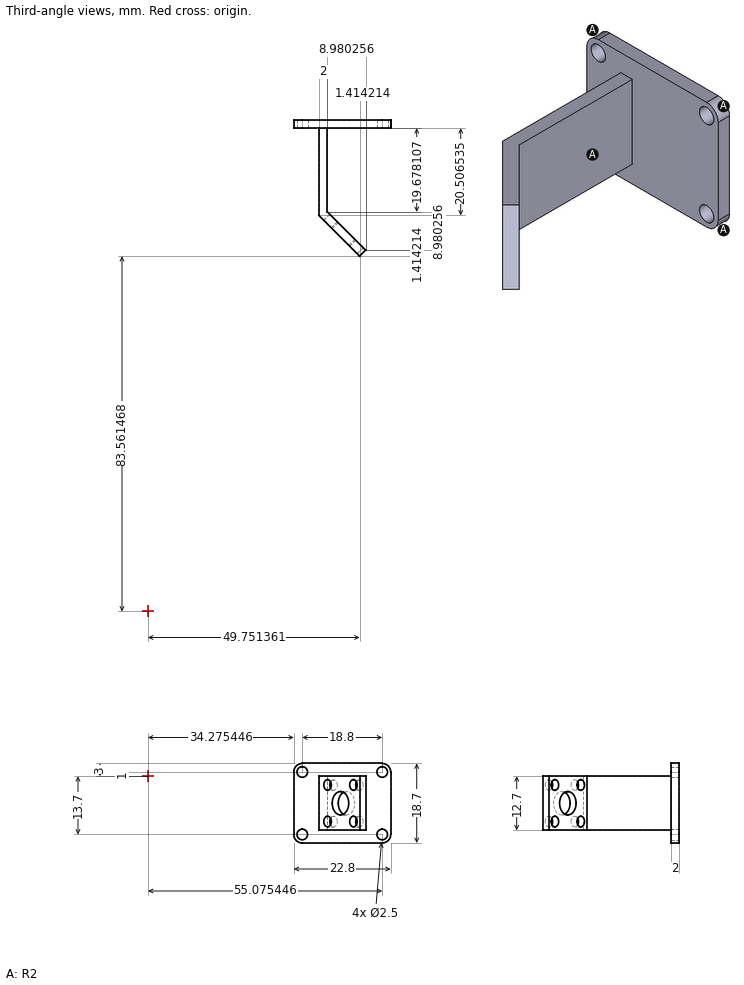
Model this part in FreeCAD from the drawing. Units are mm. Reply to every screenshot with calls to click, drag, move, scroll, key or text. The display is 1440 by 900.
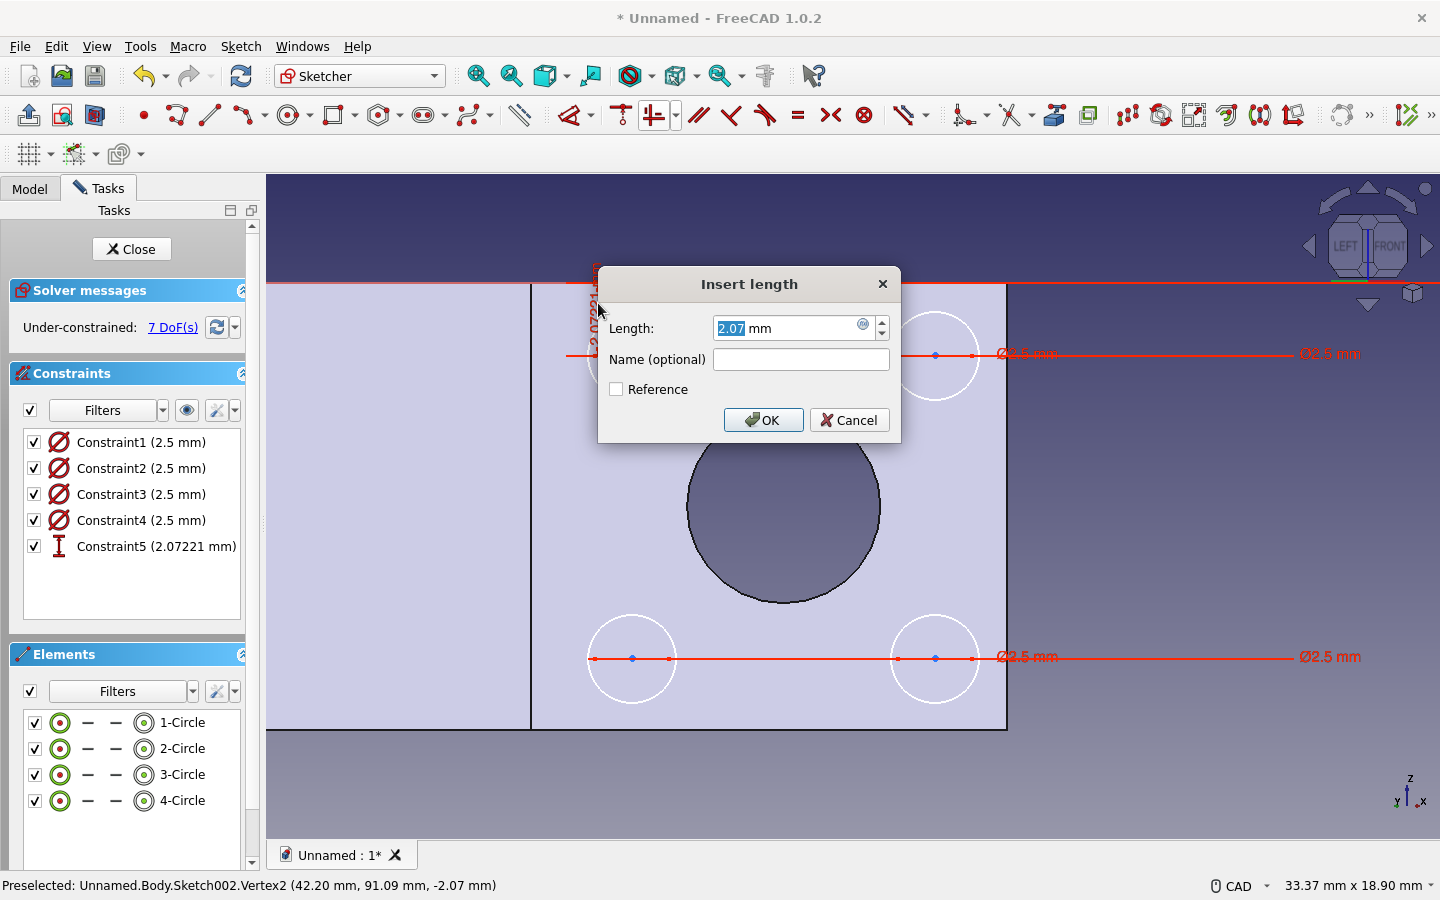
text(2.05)
key(Return)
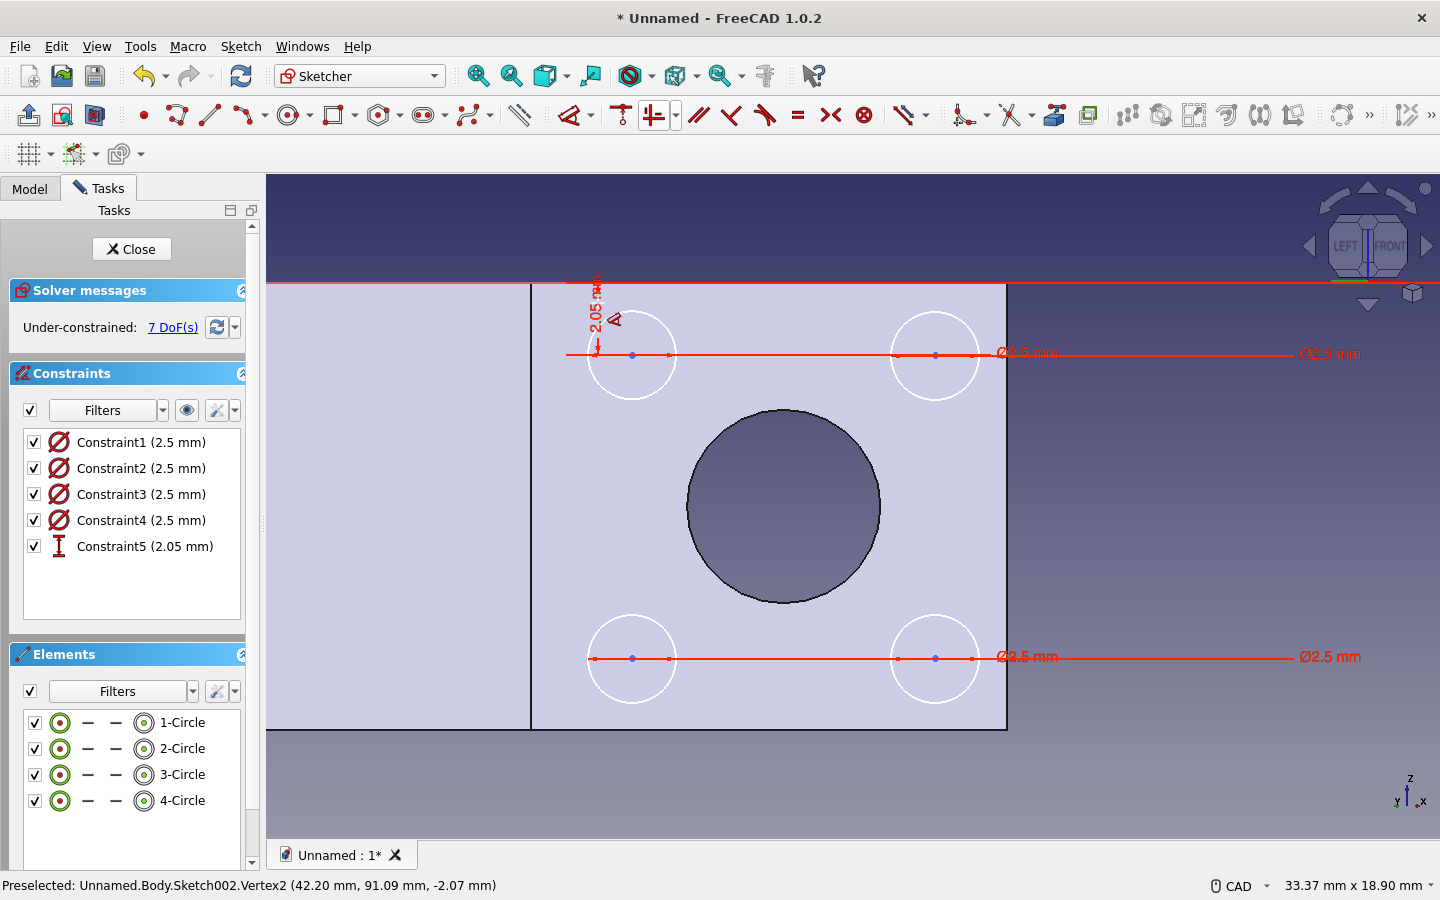
click(935, 356)
click(901, 303)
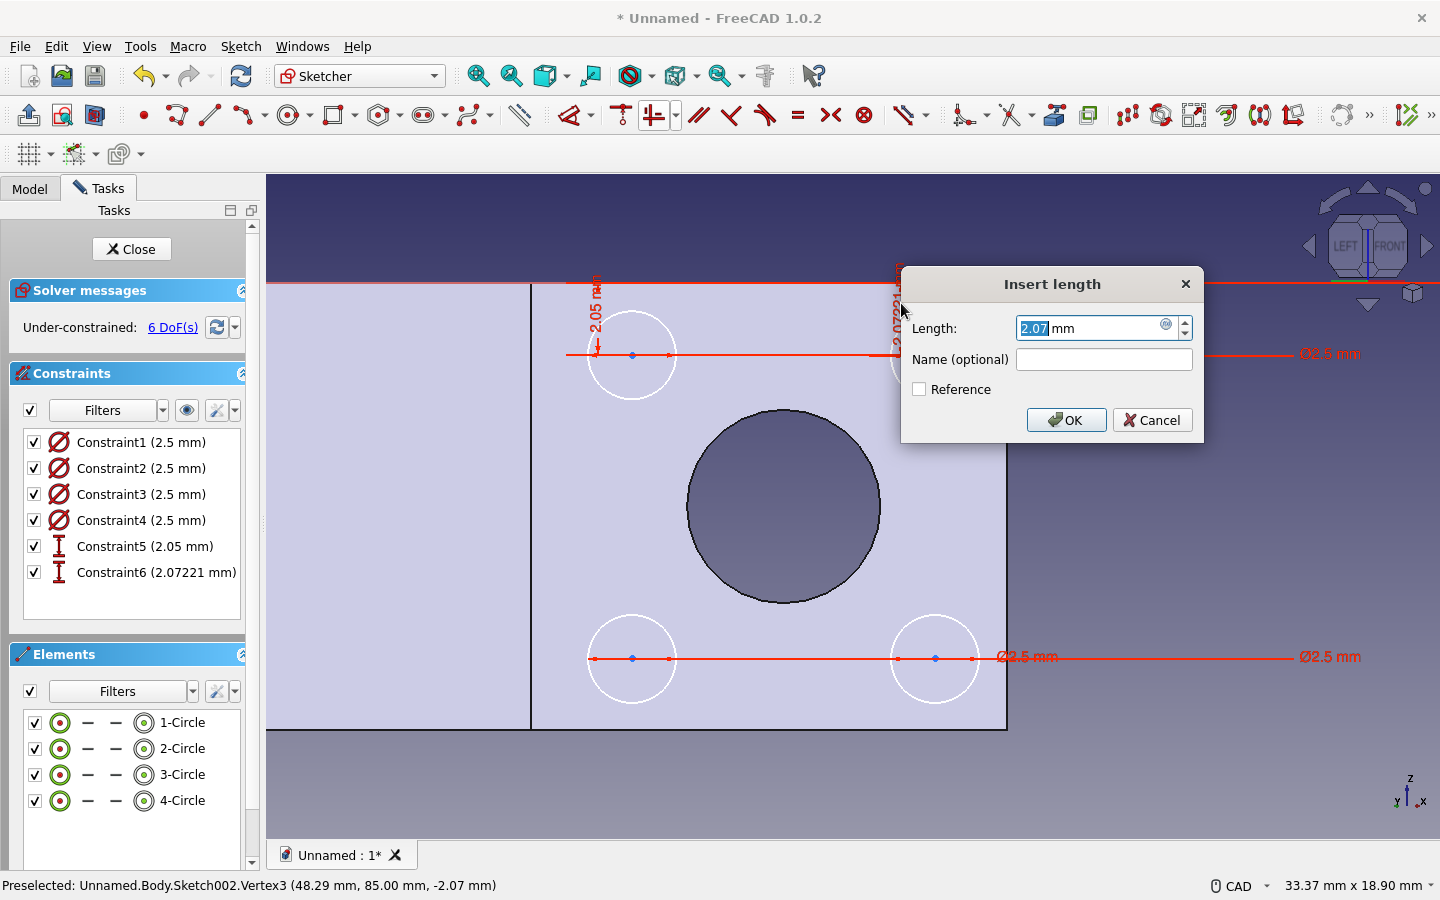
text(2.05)
key(Return)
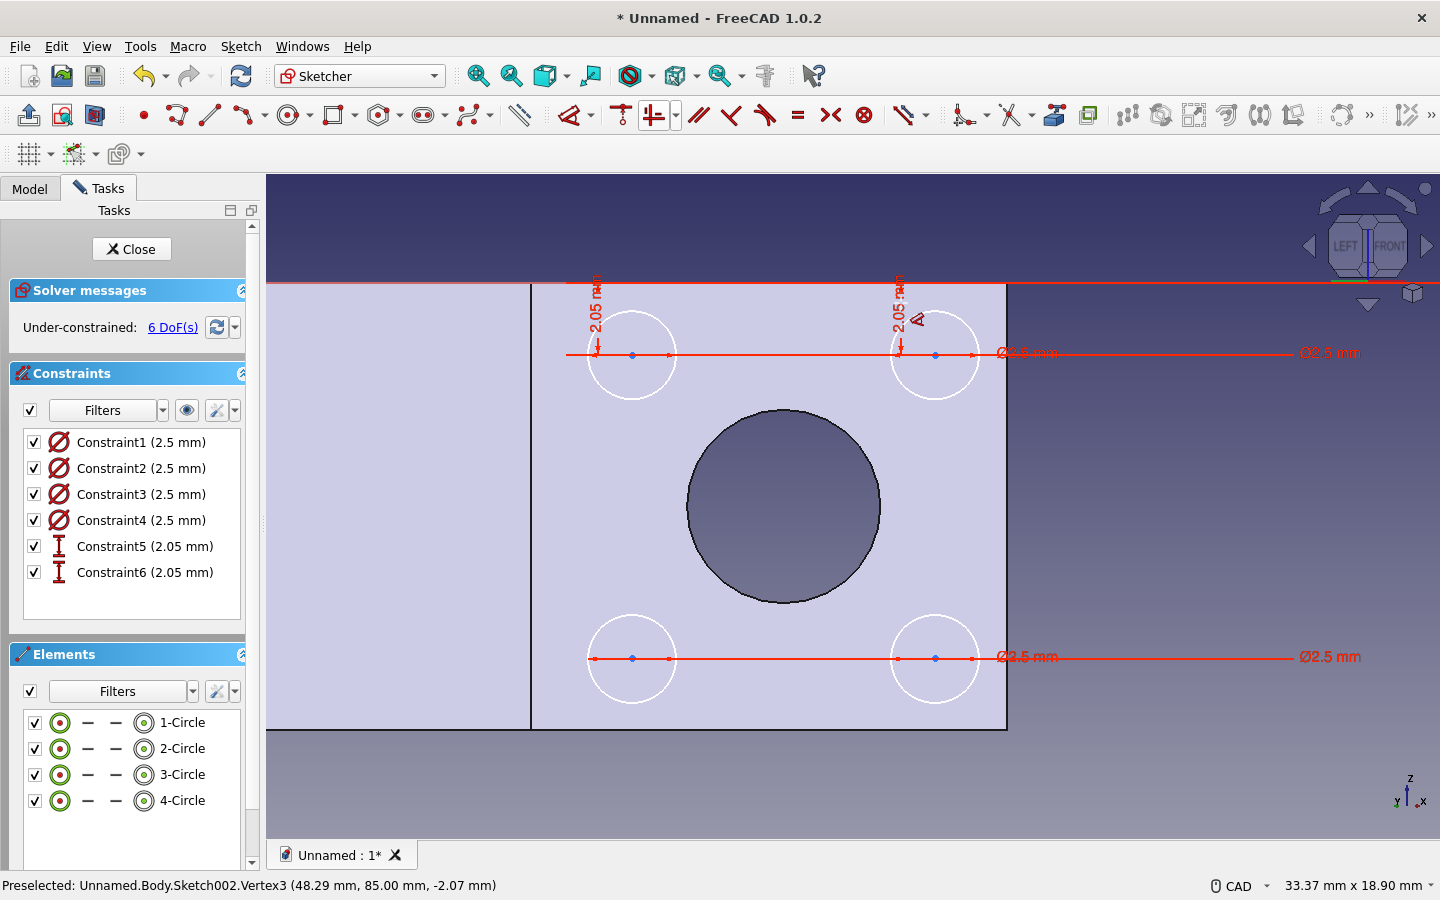
click(632, 659)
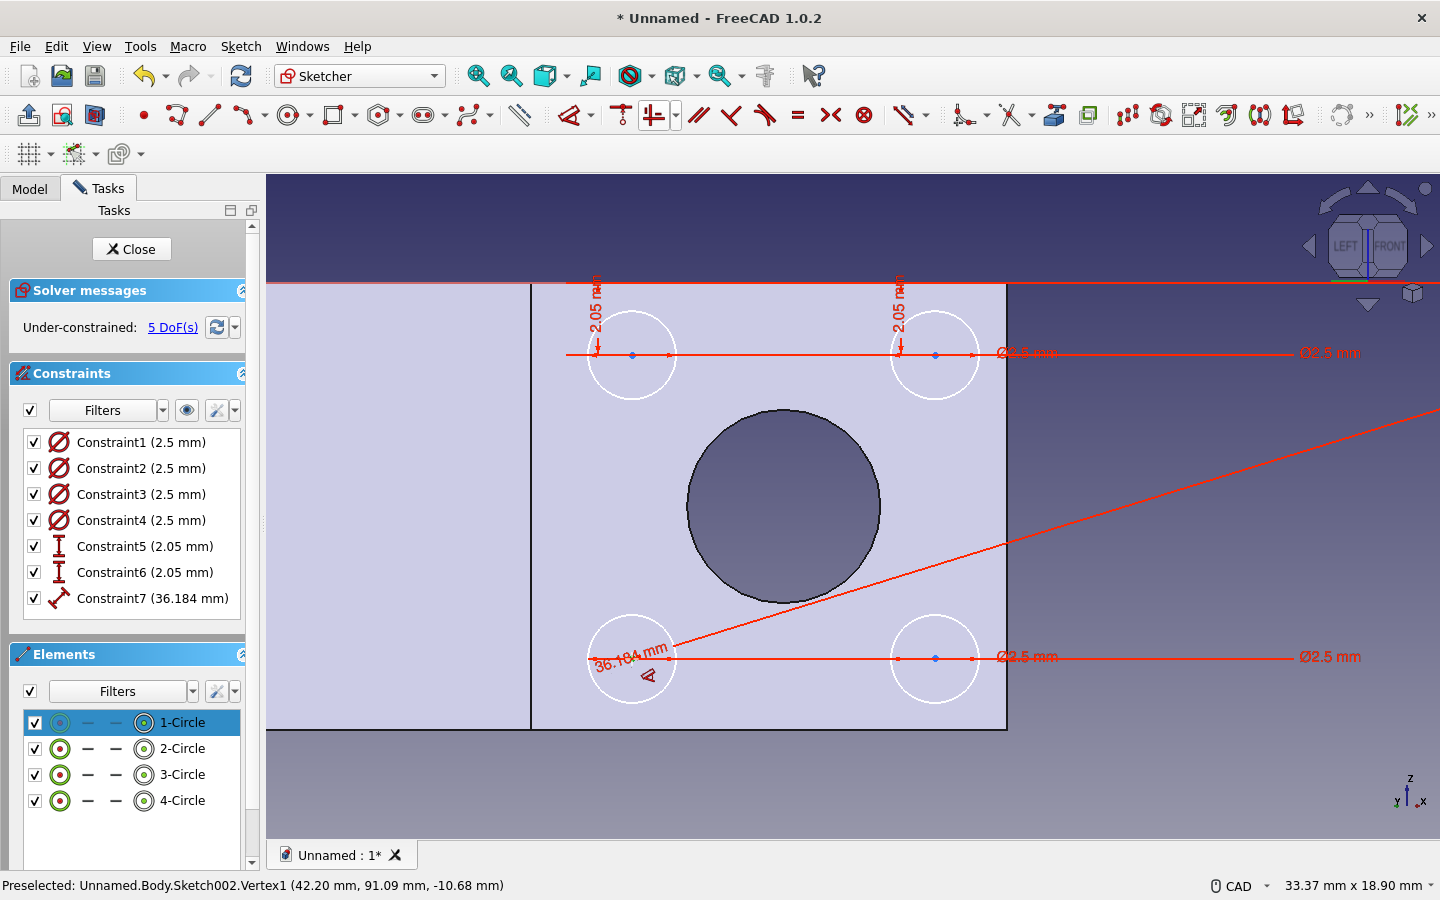
click(632, 355)
click(598, 507)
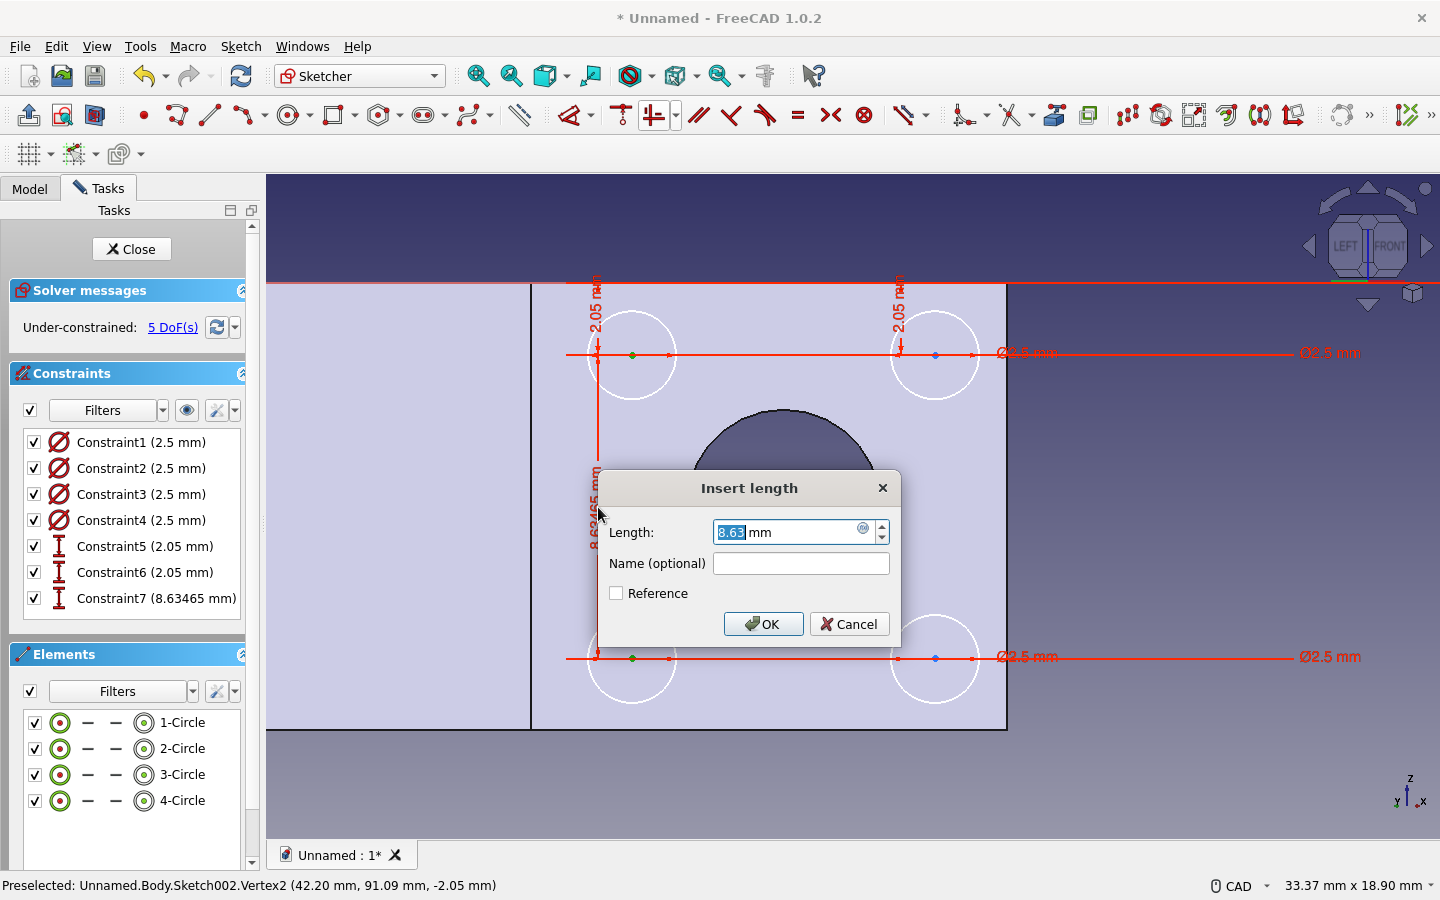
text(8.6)
key(Return)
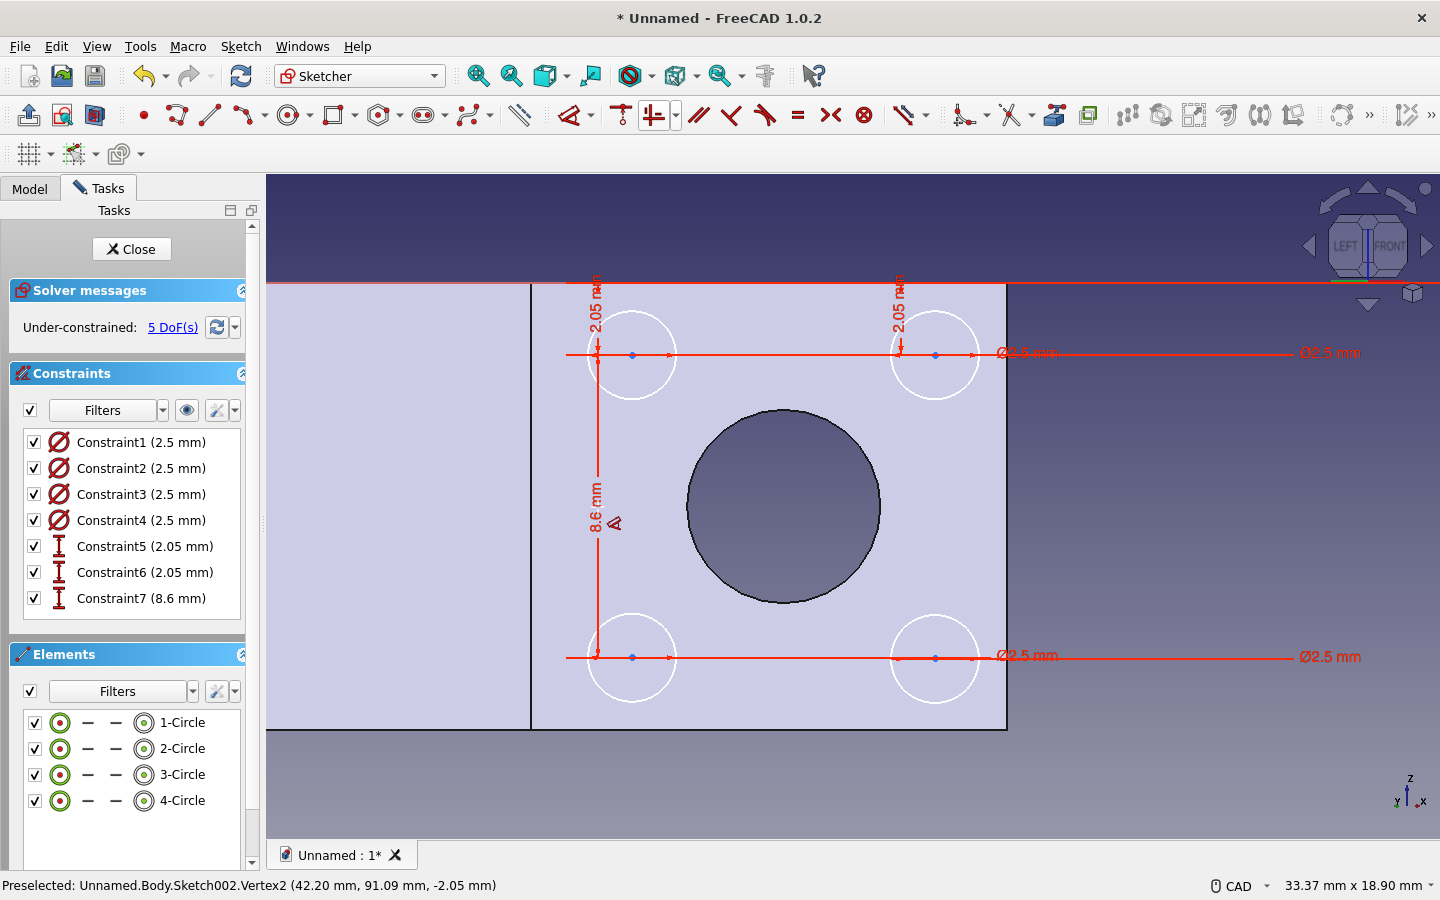
click(632, 355)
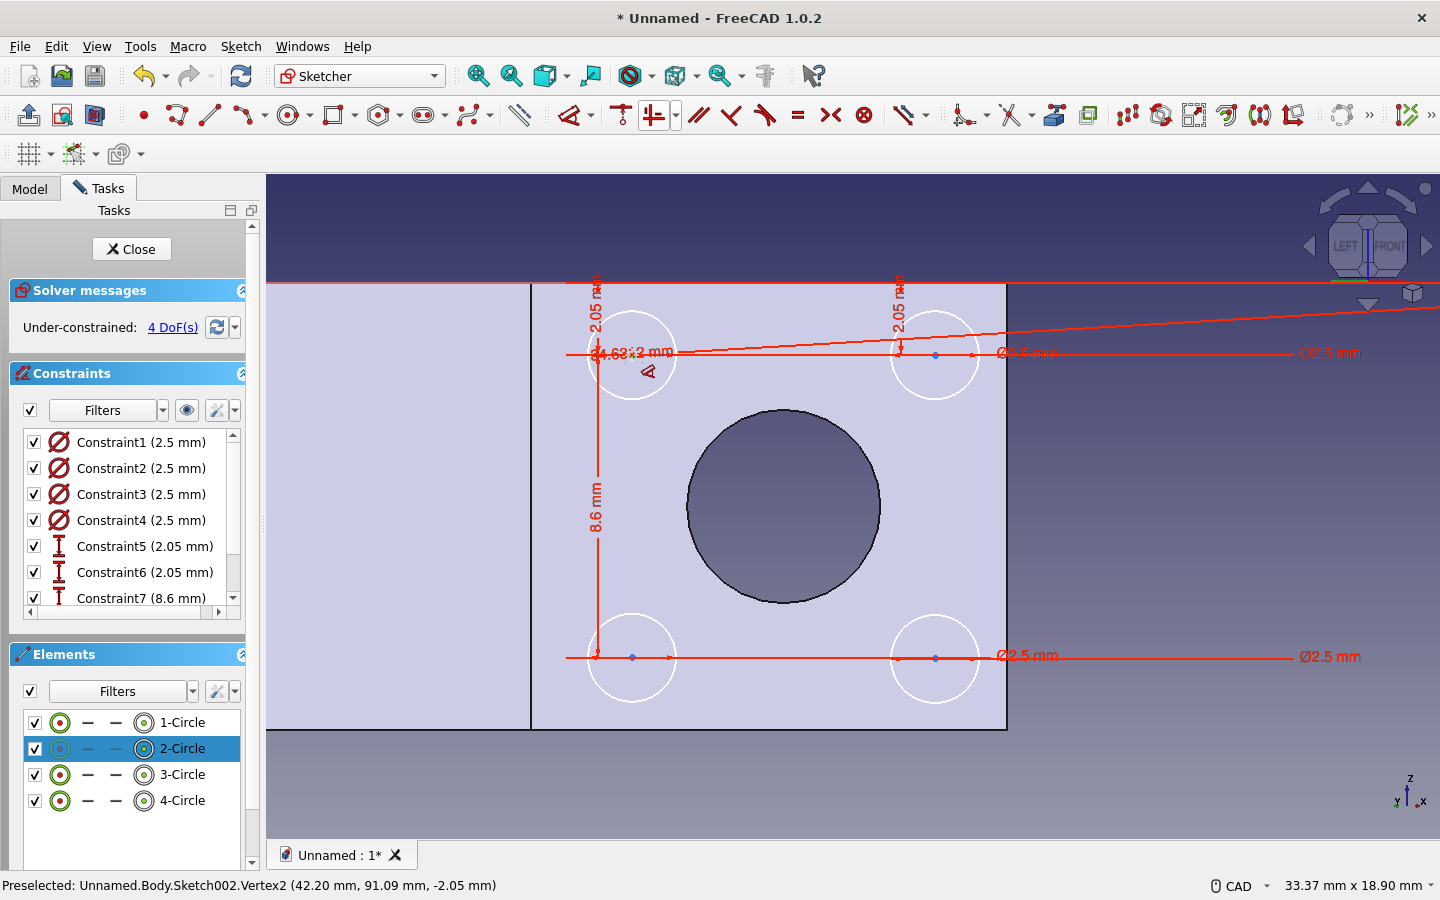
click(935, 355)
click(784, 321)